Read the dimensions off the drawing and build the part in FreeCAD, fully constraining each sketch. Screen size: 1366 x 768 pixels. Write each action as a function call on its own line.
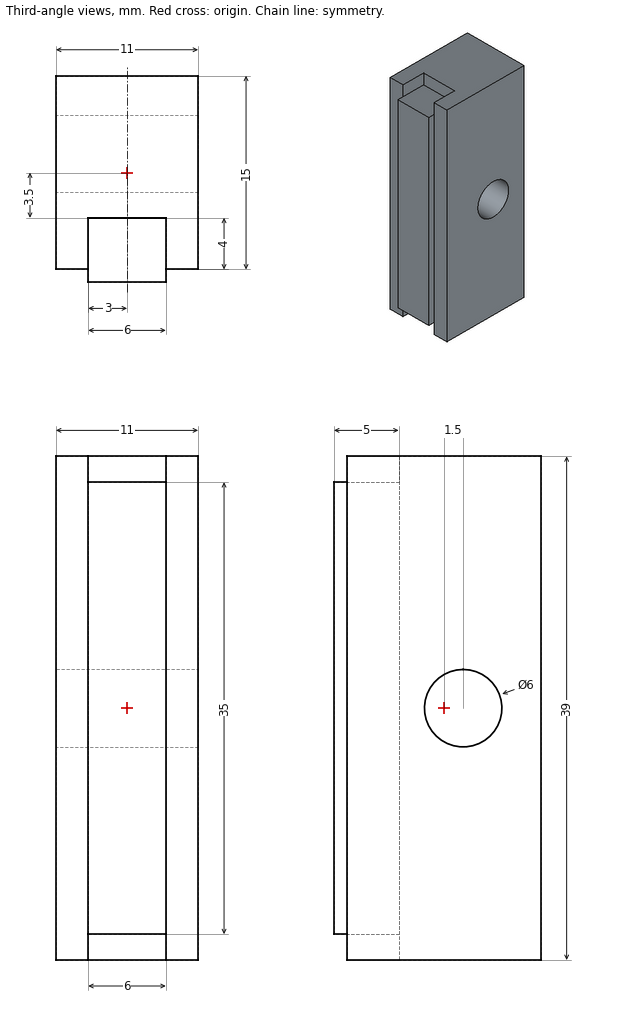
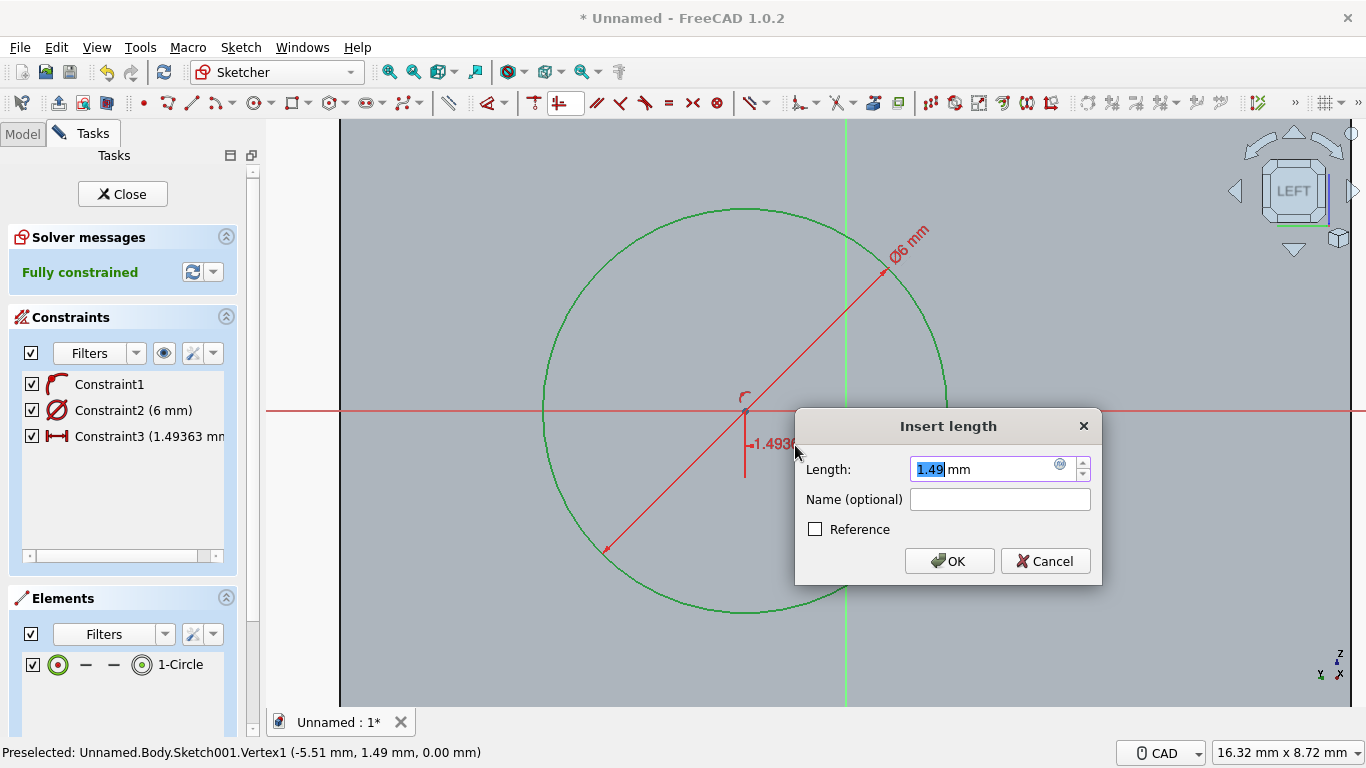
text(1.5)
key(Return)
key(Escape)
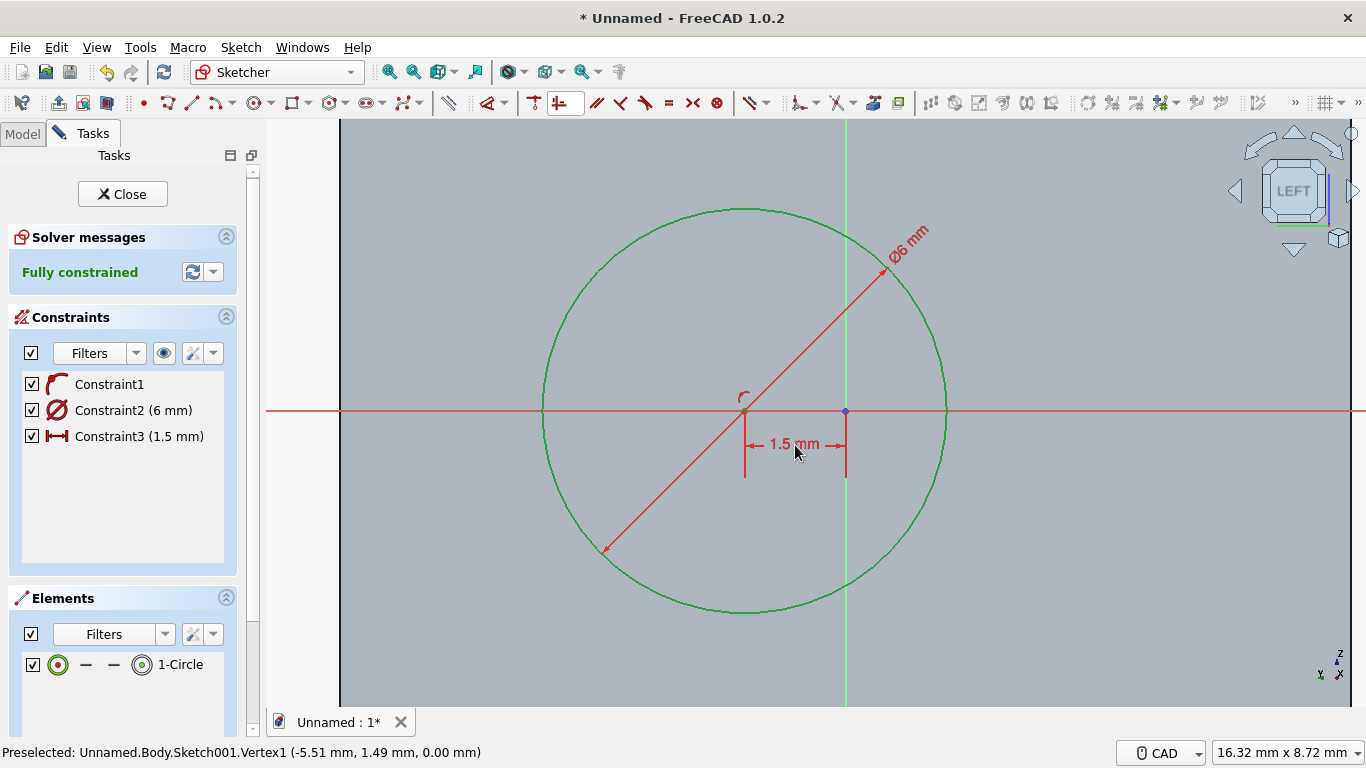
click(123, 194)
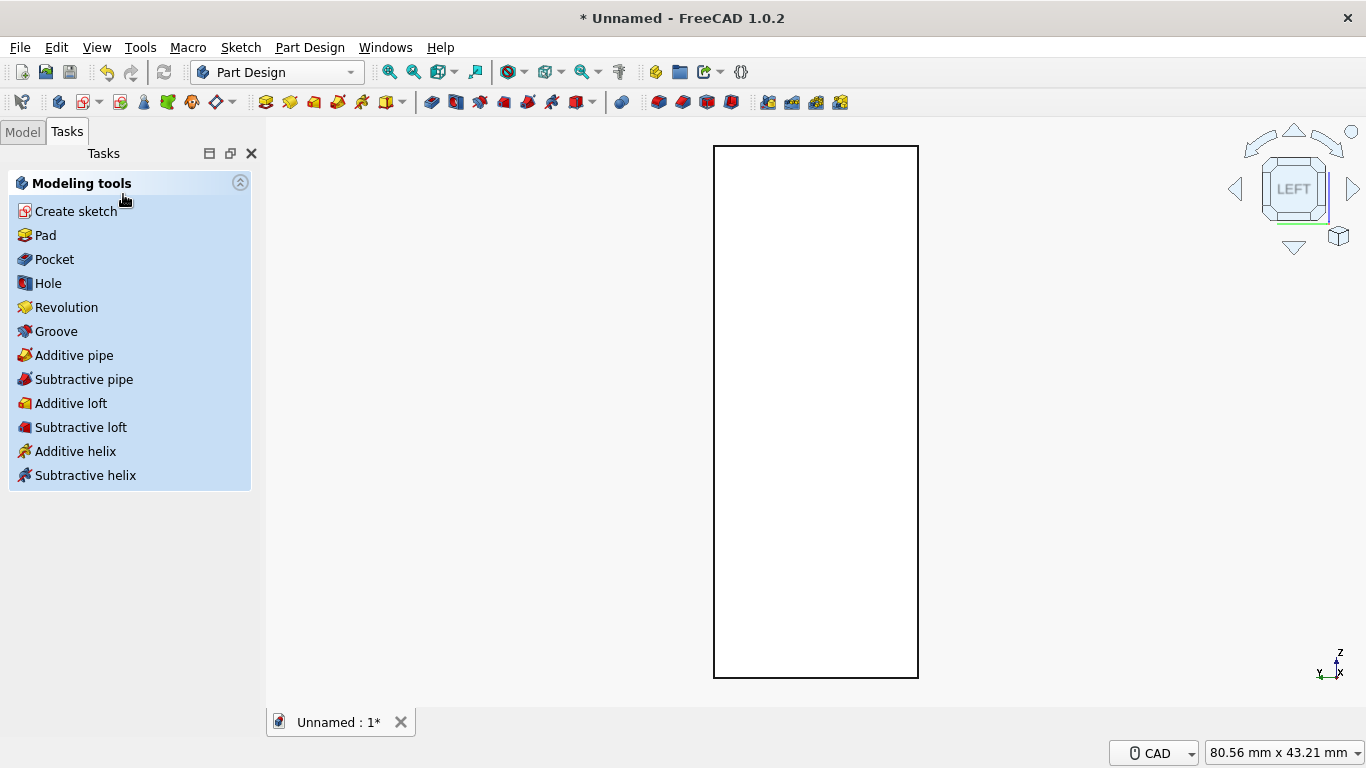
click(432, 102)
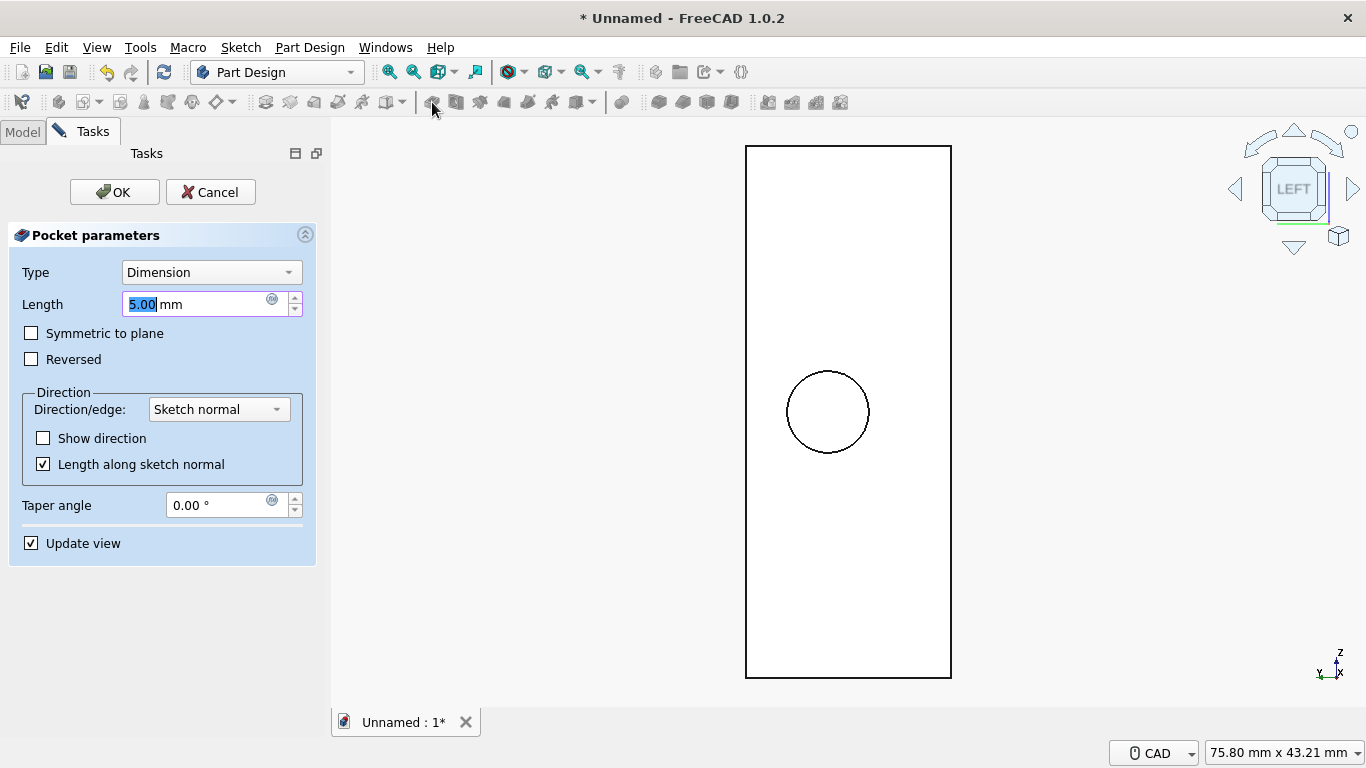
text(11)
key(Tab)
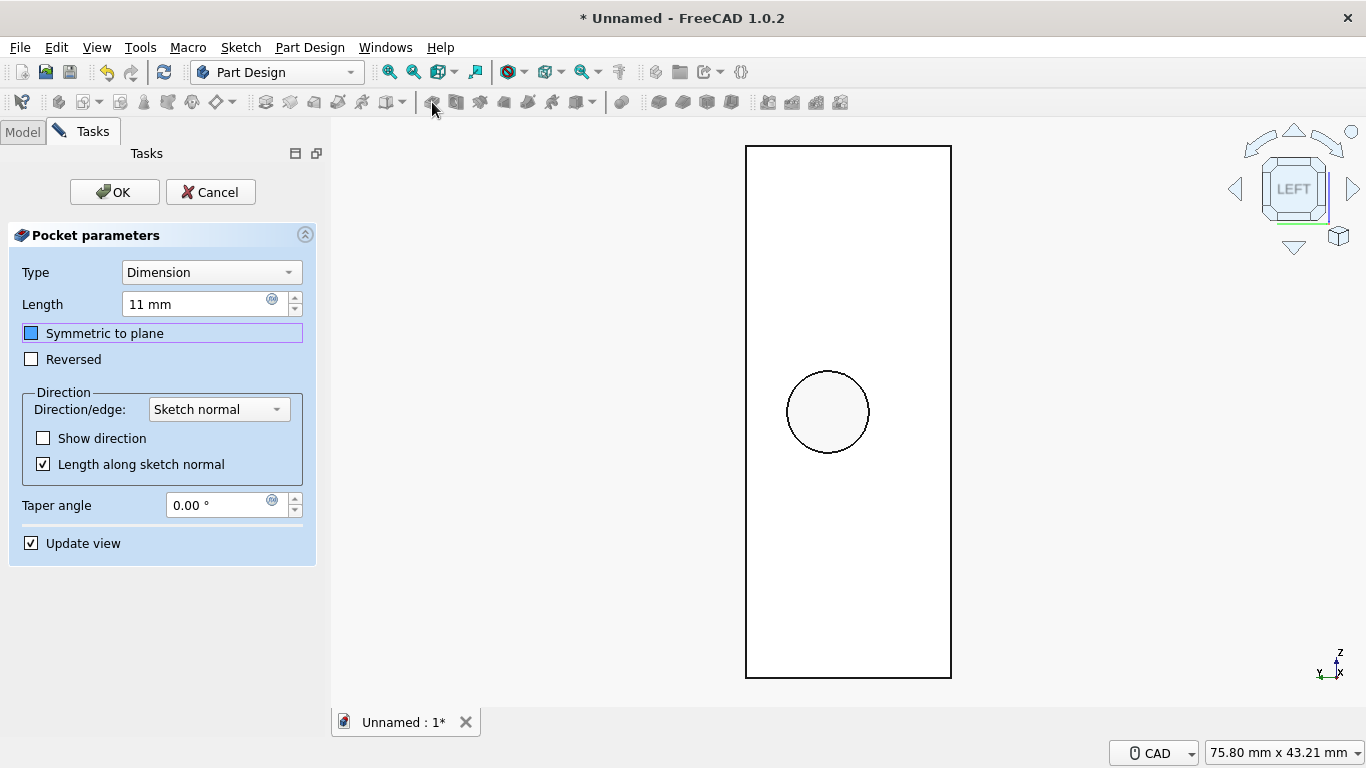
click(115, 192)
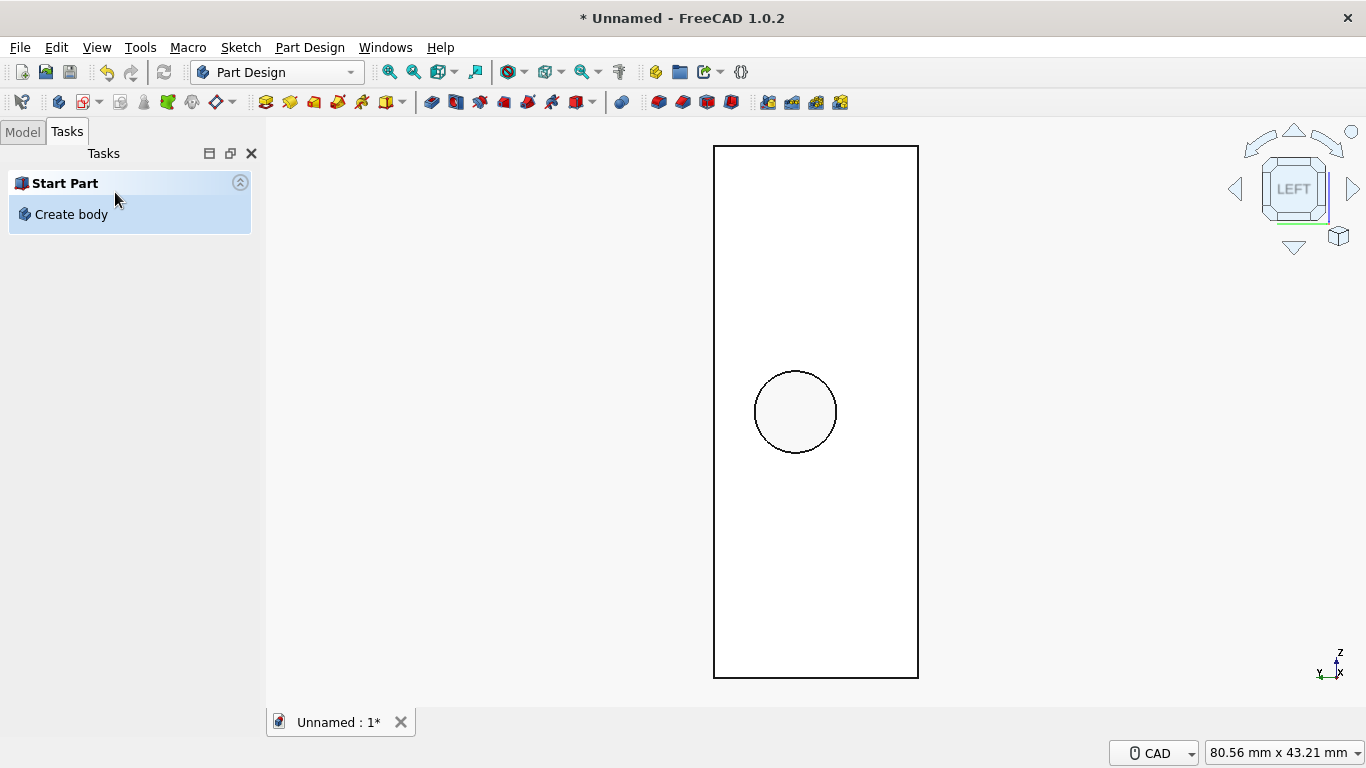
click(60, 102)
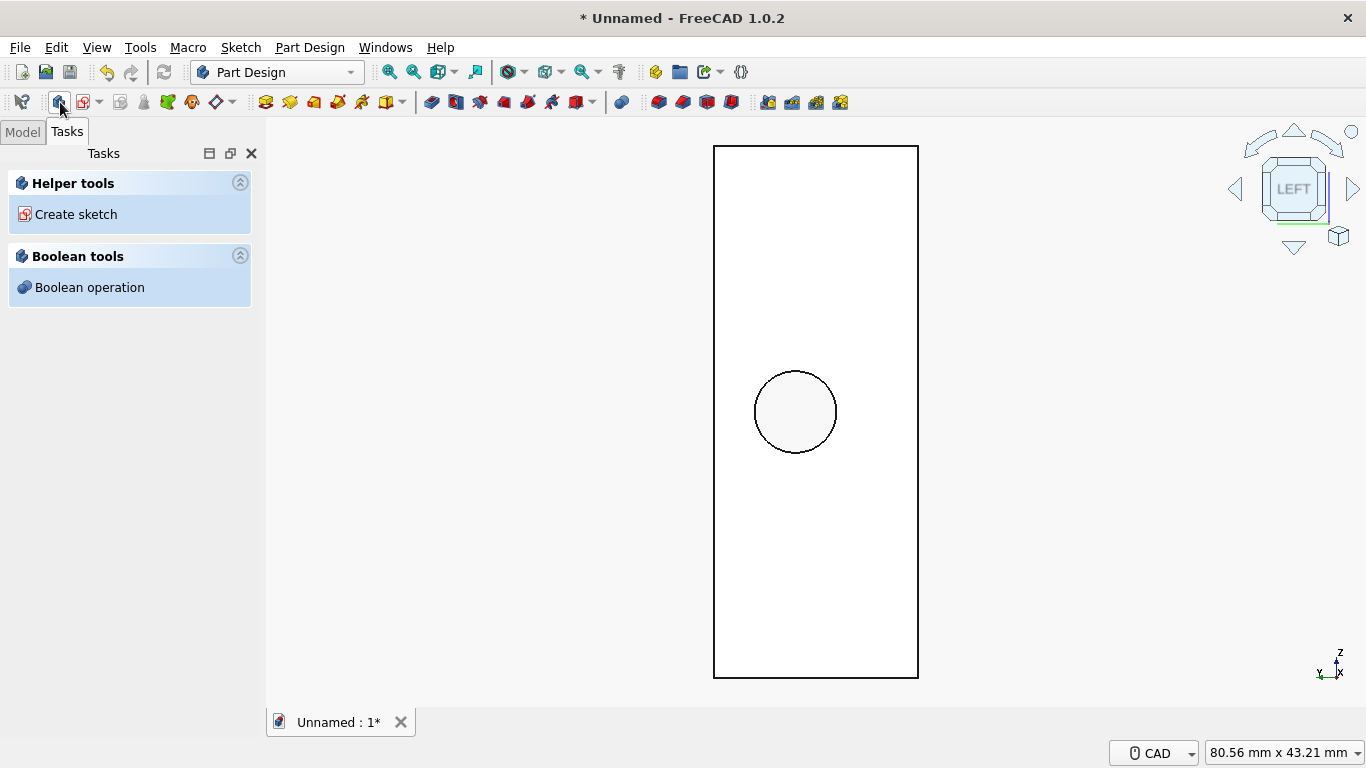
click(23, 131)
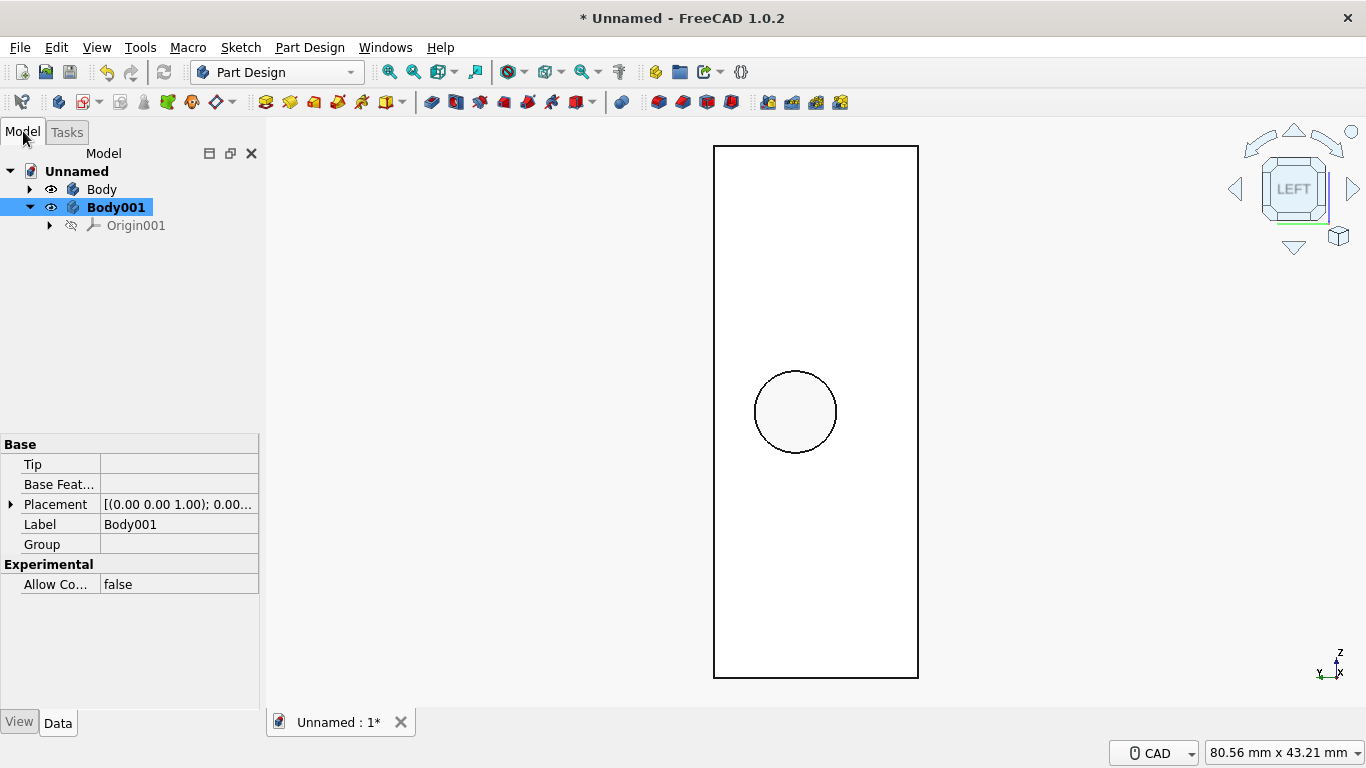
click(50, 225)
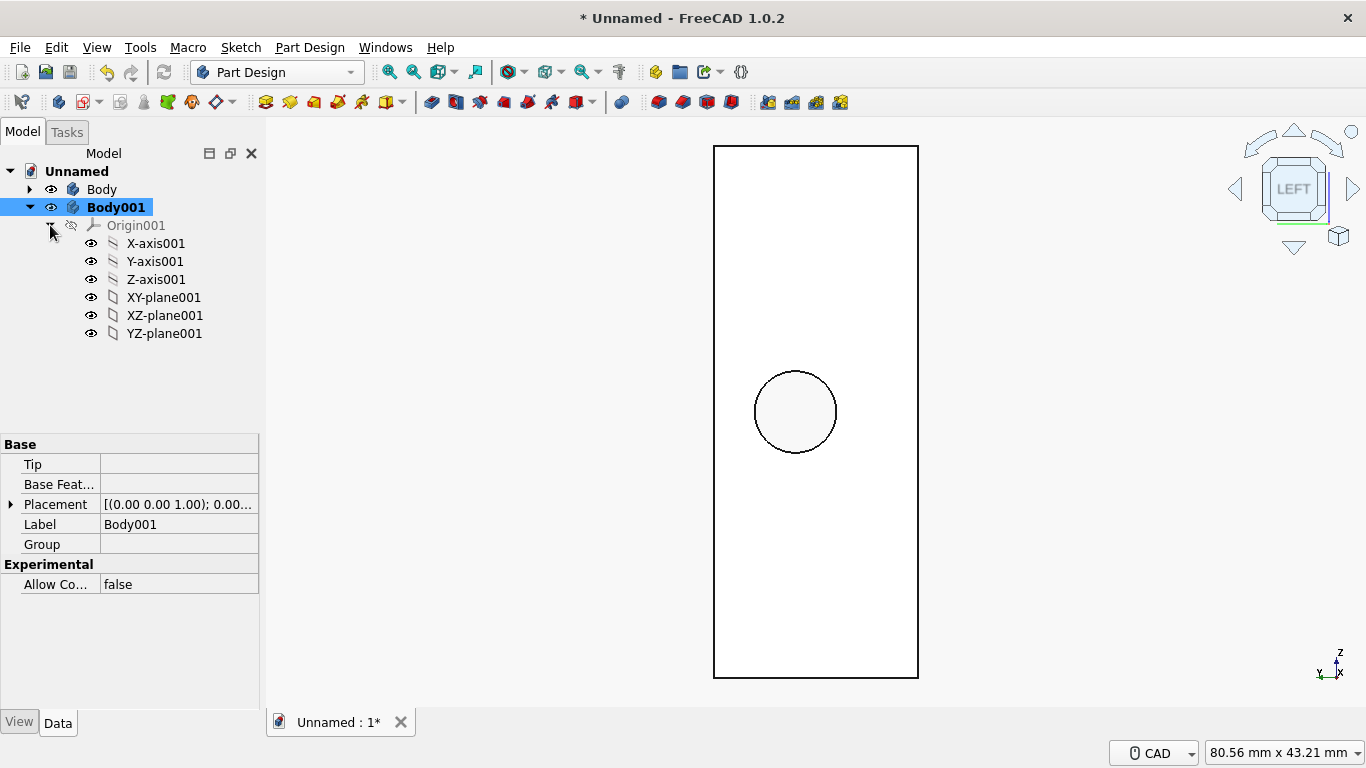
click(136, 315)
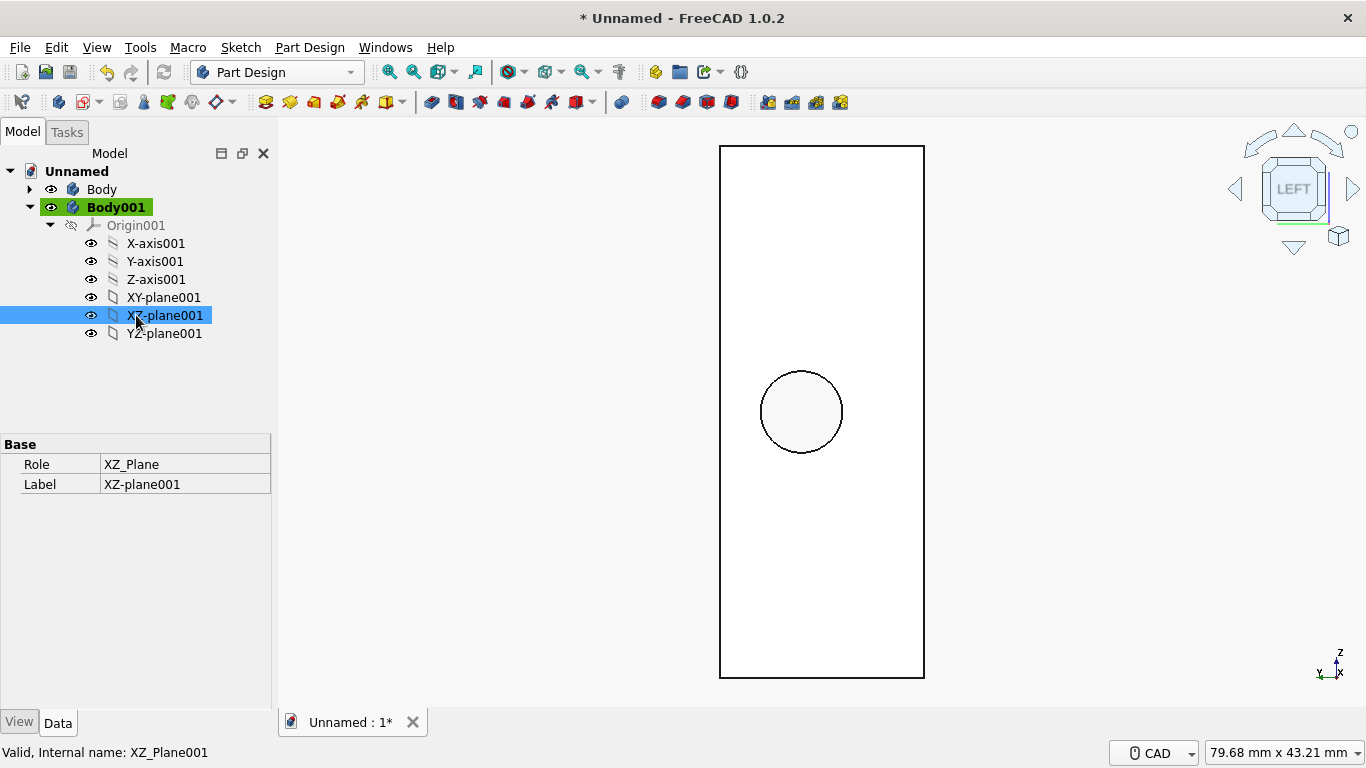
click(216, 102)